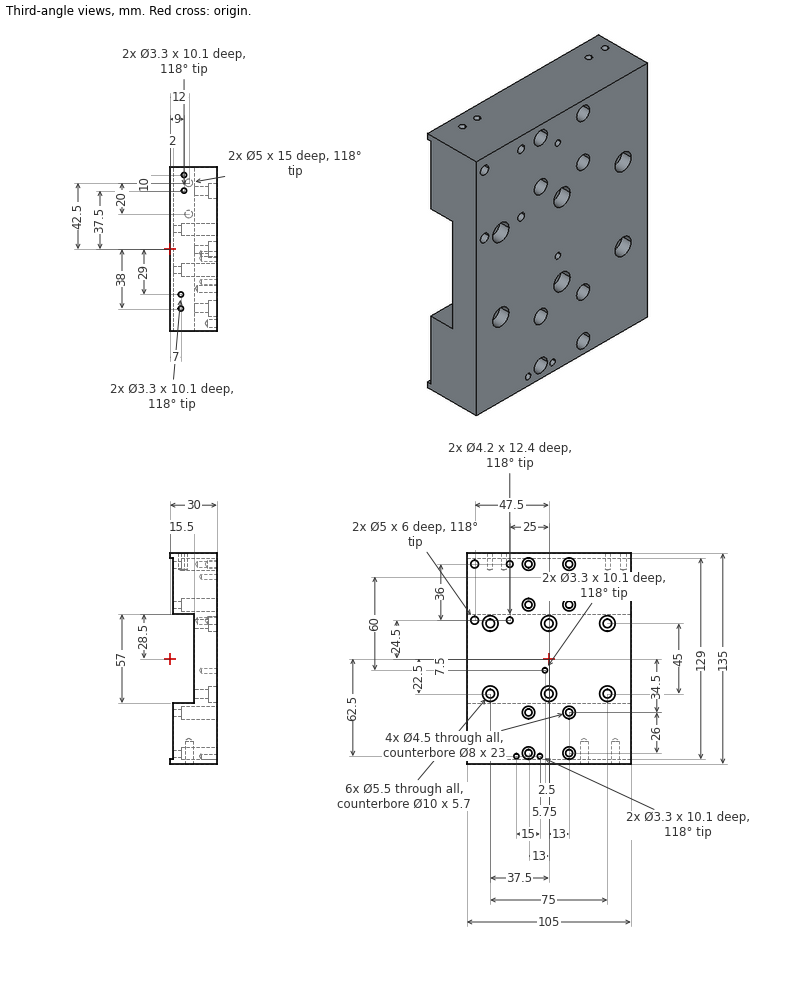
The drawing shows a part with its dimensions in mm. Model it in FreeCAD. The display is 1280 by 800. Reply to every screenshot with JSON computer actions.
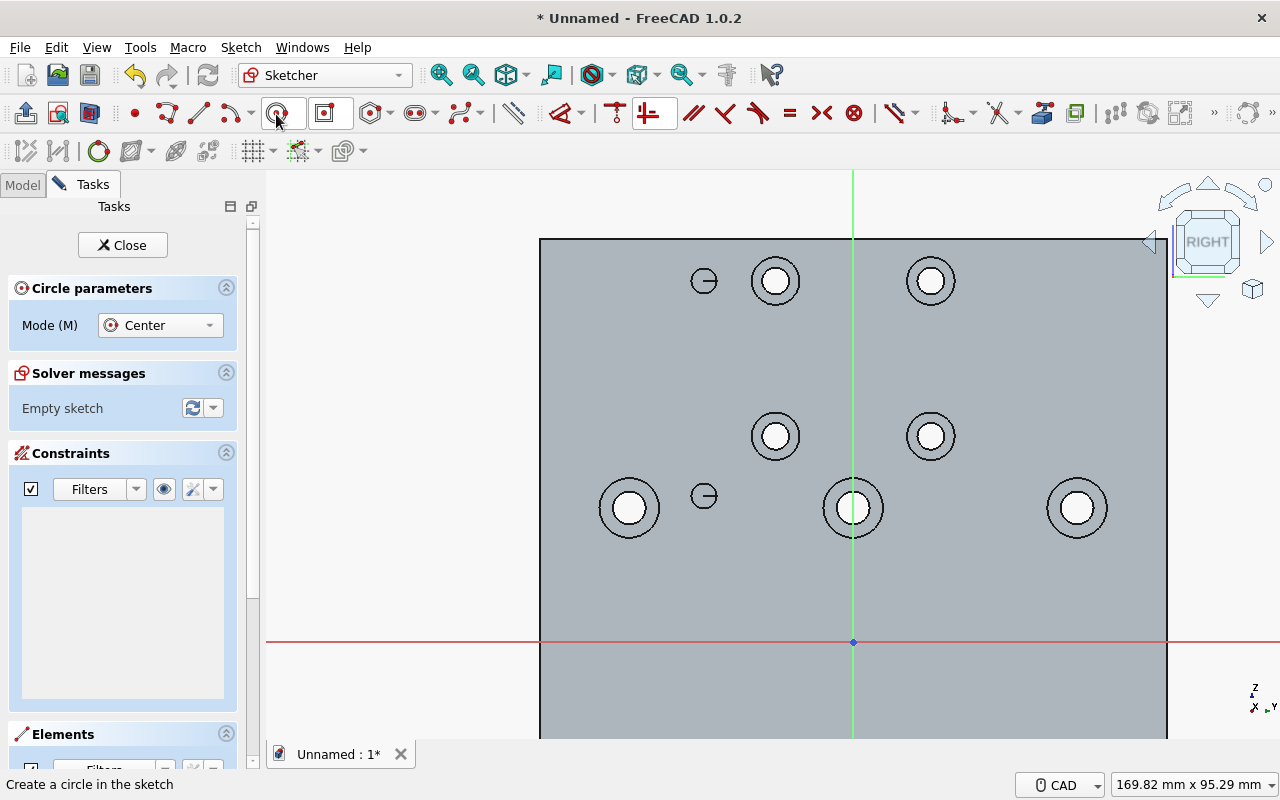
{"action": "scroll", "coordinate": [570, 496], "scroll_direction": "up", "scroll_amount": 3}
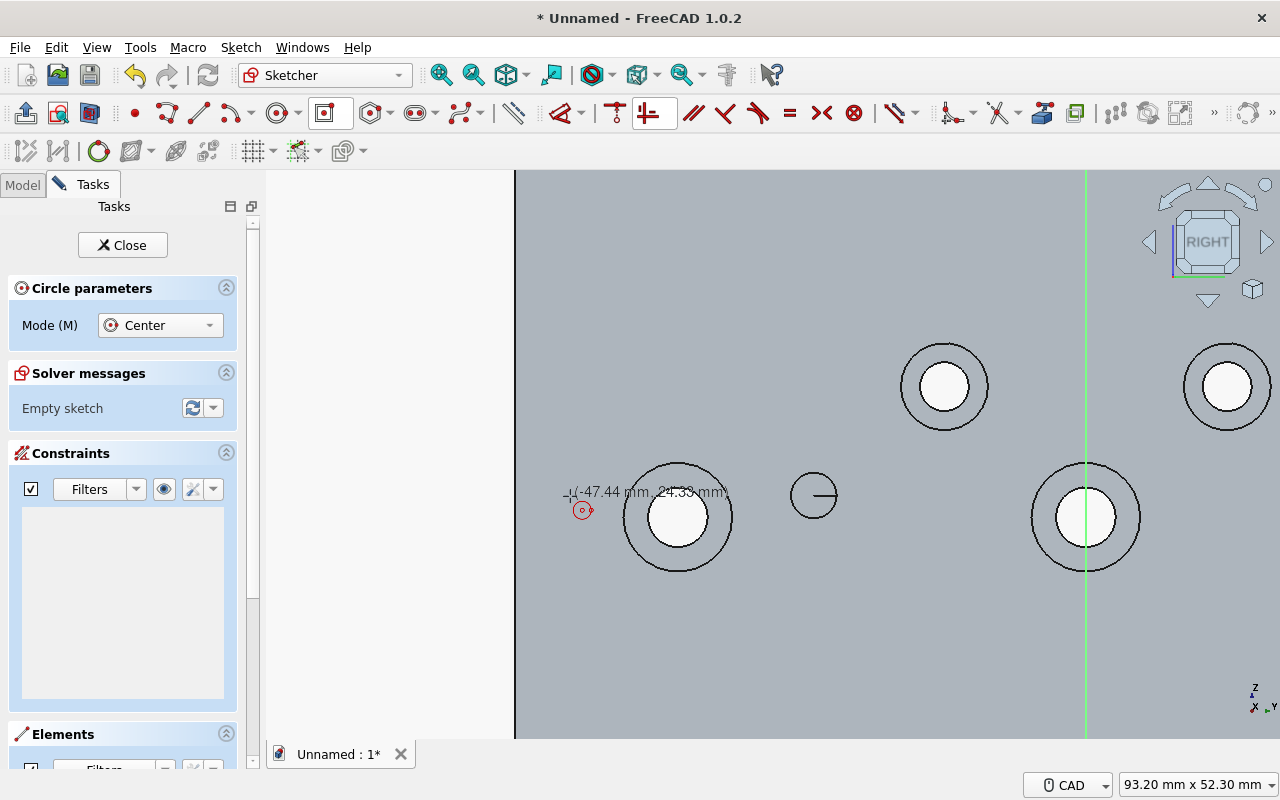
{"action": "left_click", "coordinate": [569, 495]}
{"action": "left_click", "coordinate": [588, 476]}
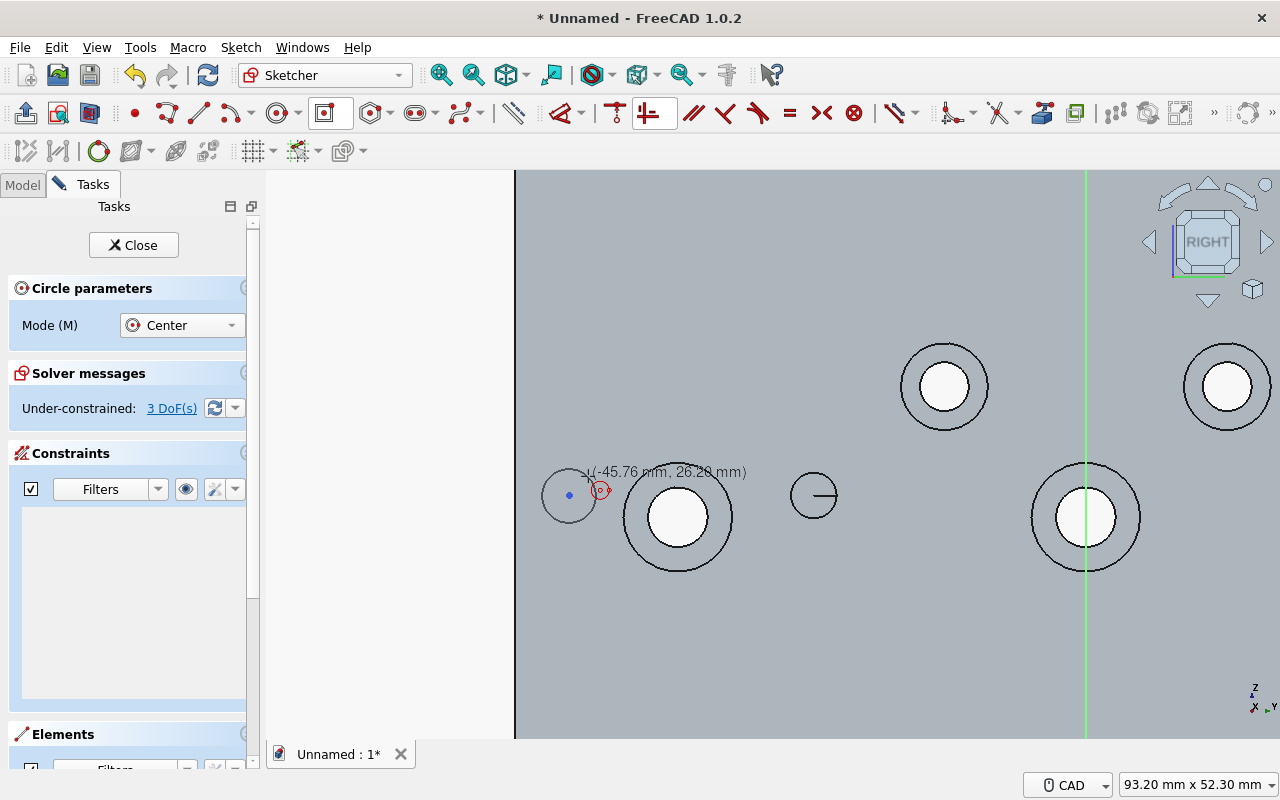
{"action": "scroll", "coordinate": [571, 497], "scroll_direction": "down", "scroll_amount": 3}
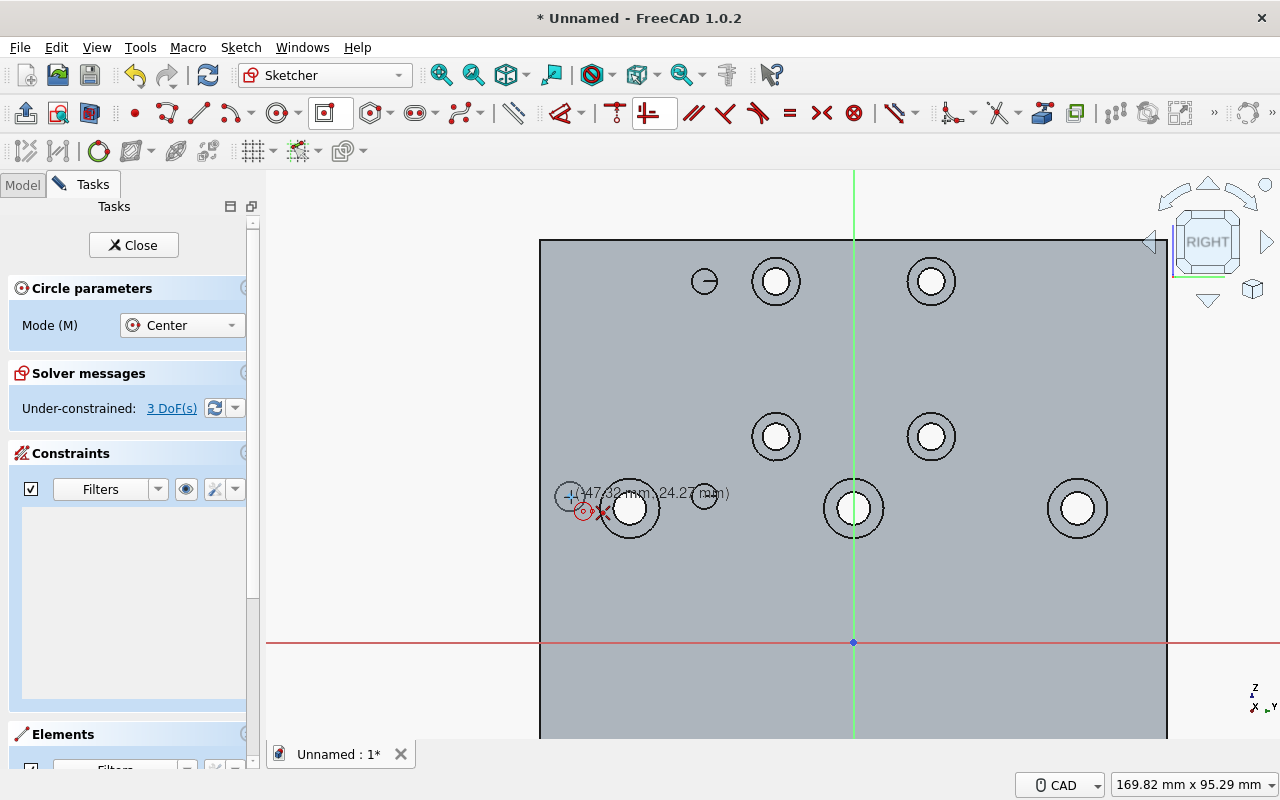
{"action": "scroll", "coordinate": [570, 281], "scroll_direction": "up", "scroll_amount": 3}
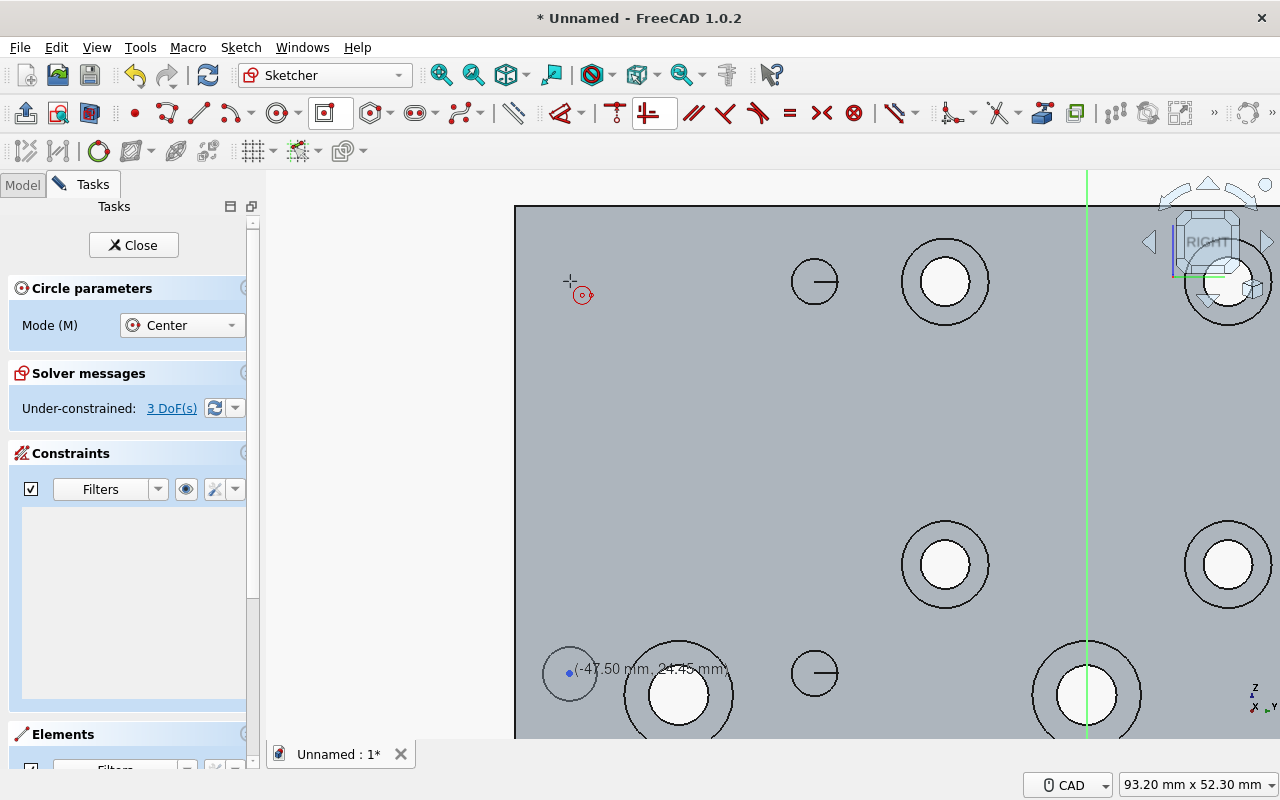
{"action": "left_click", "coordinate": [570, 282]}
{"action": "left_click", "coordinate": [589, 262]}
{"action": "key", "text": "Escape"}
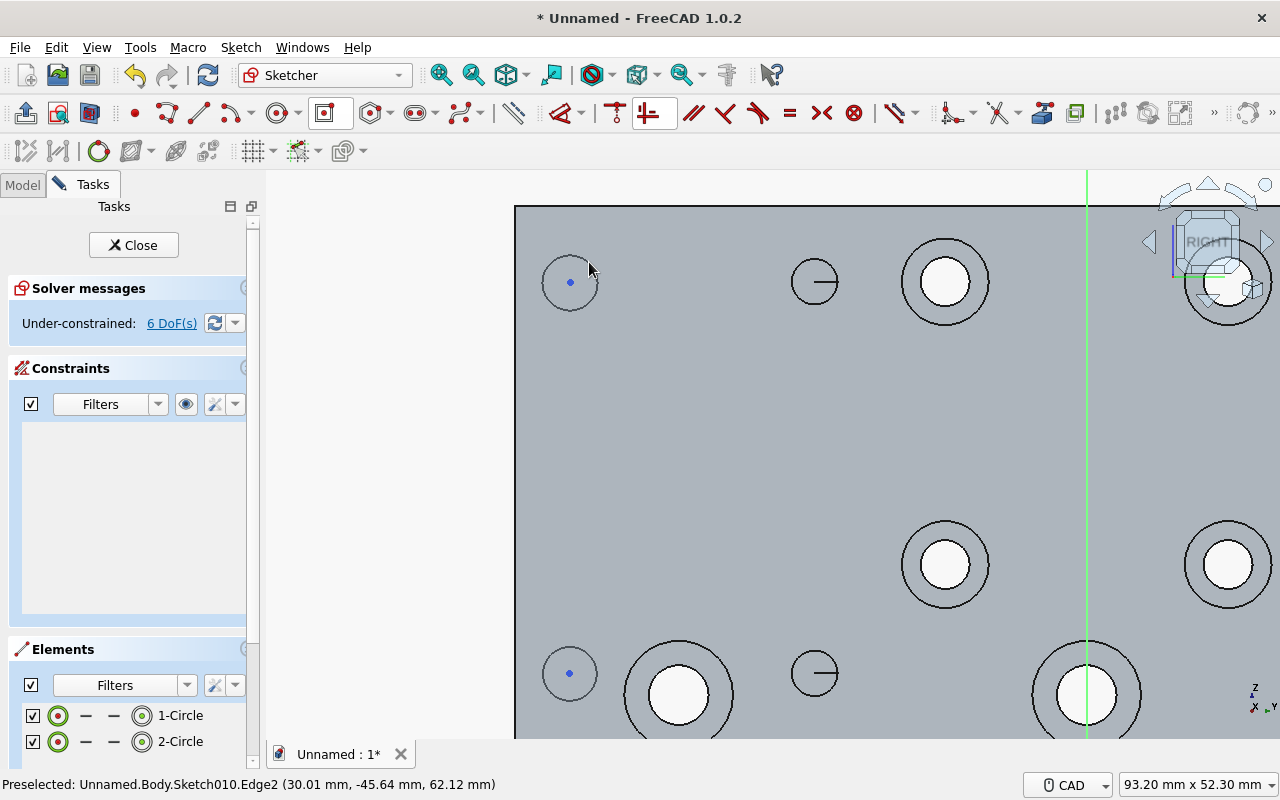
{"action": "left_click", "coordinate": [589, 655]}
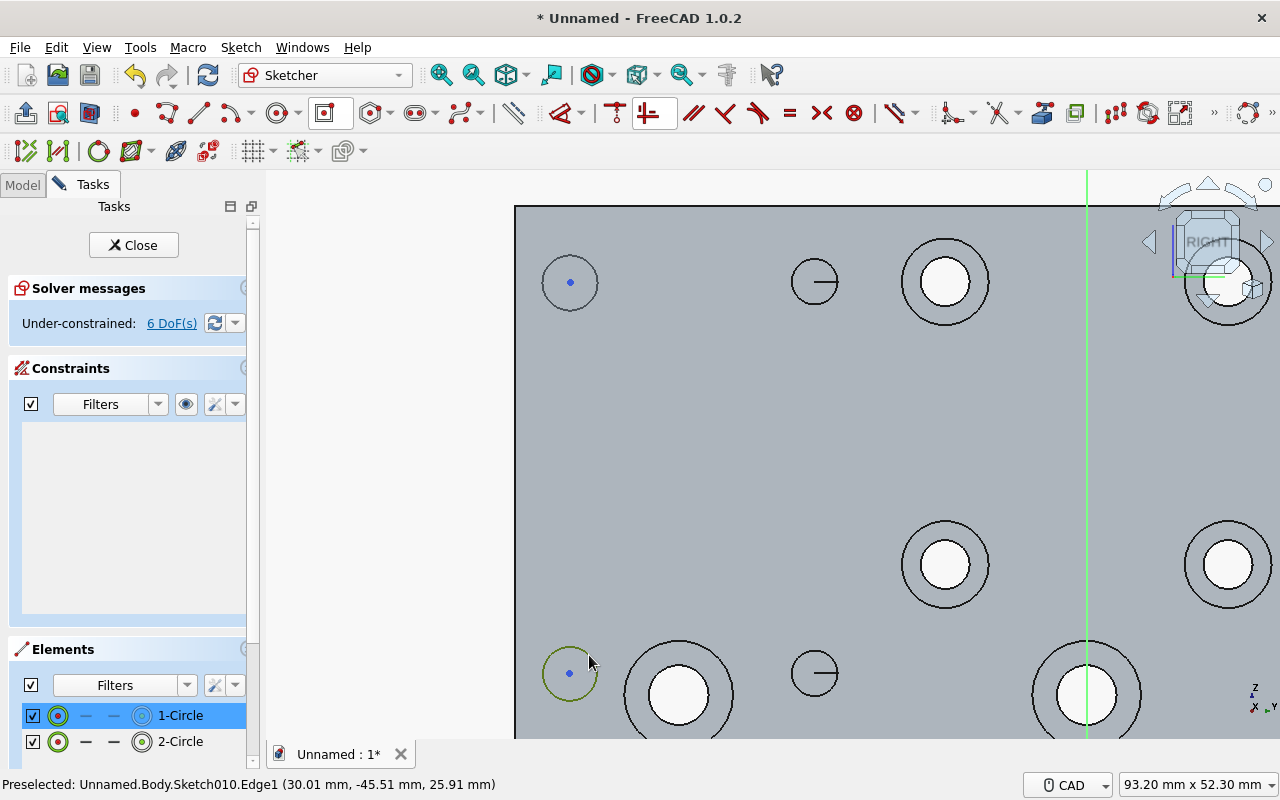
{"action": "left_click", "coordinate": [589, 263]}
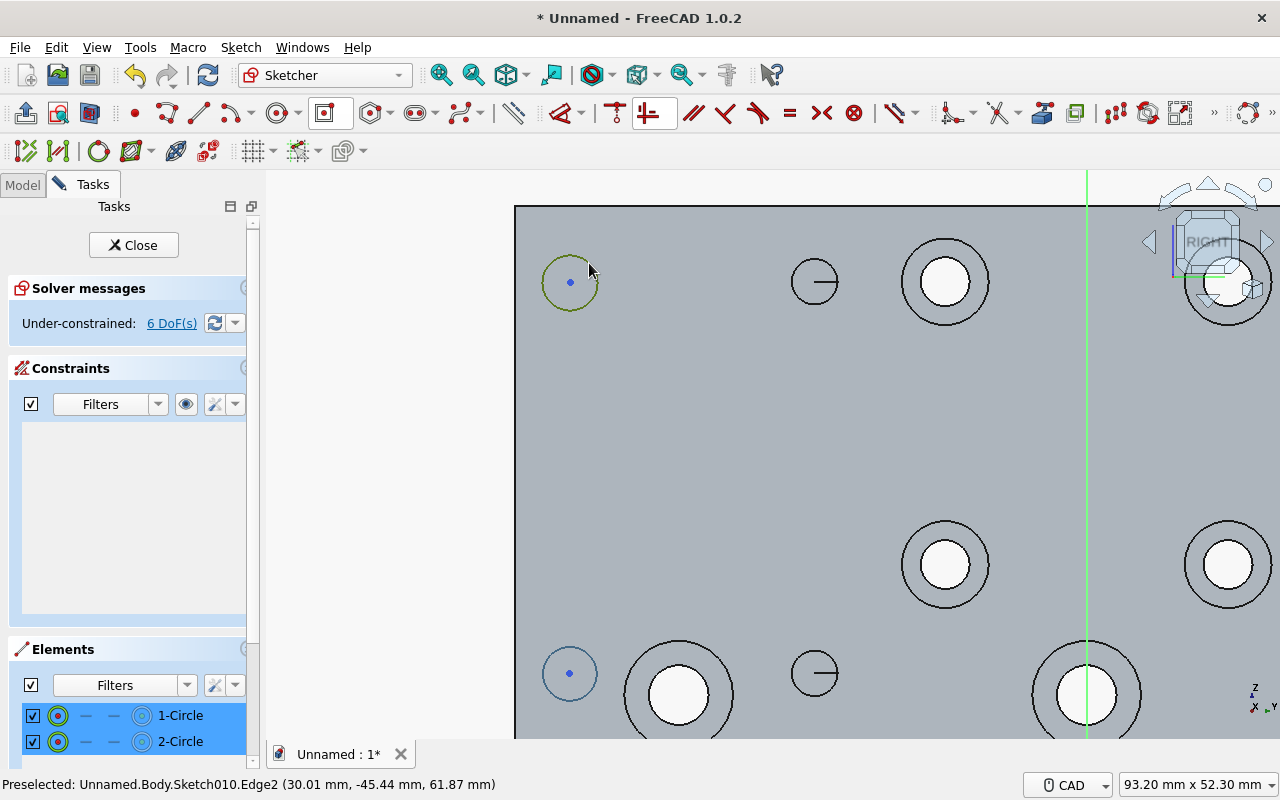
{"action": "left_click", "coordinate": [790, 114]}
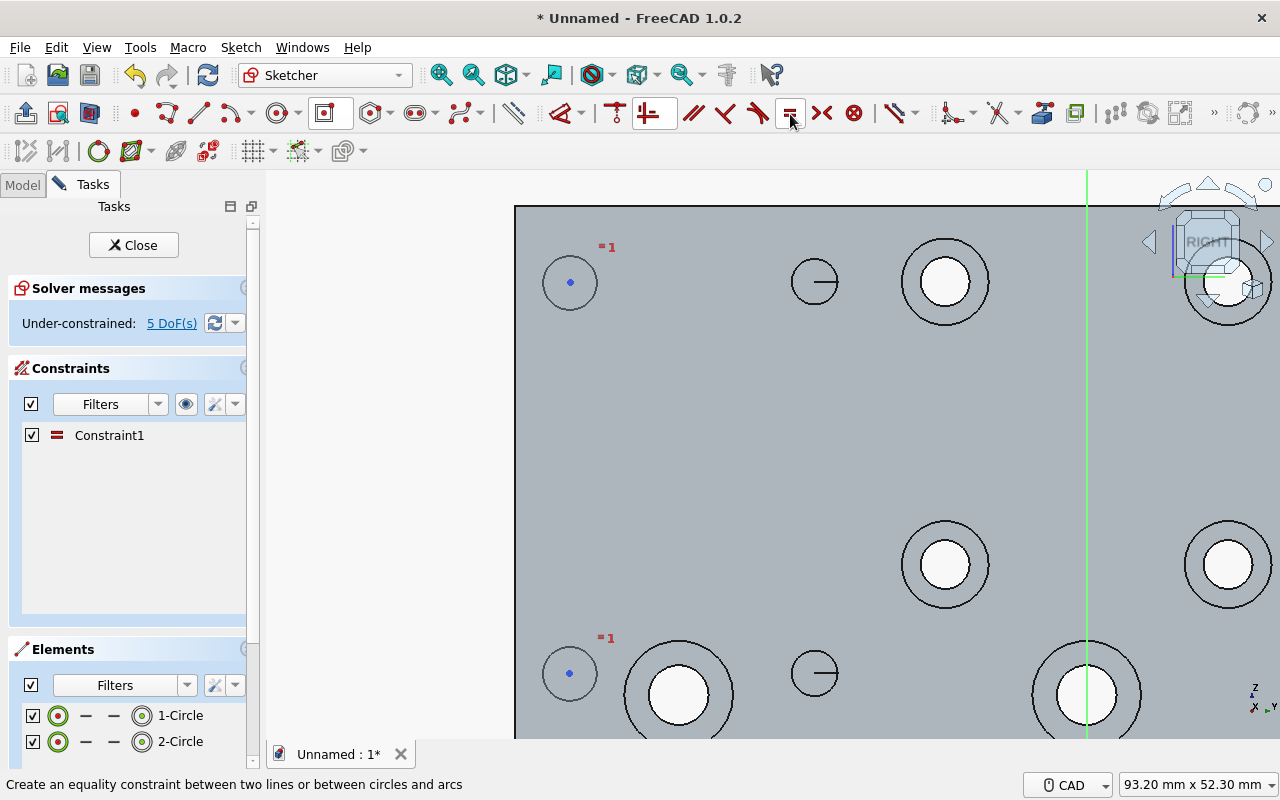
{"action": "left_click", "coordinate": [570, 674]}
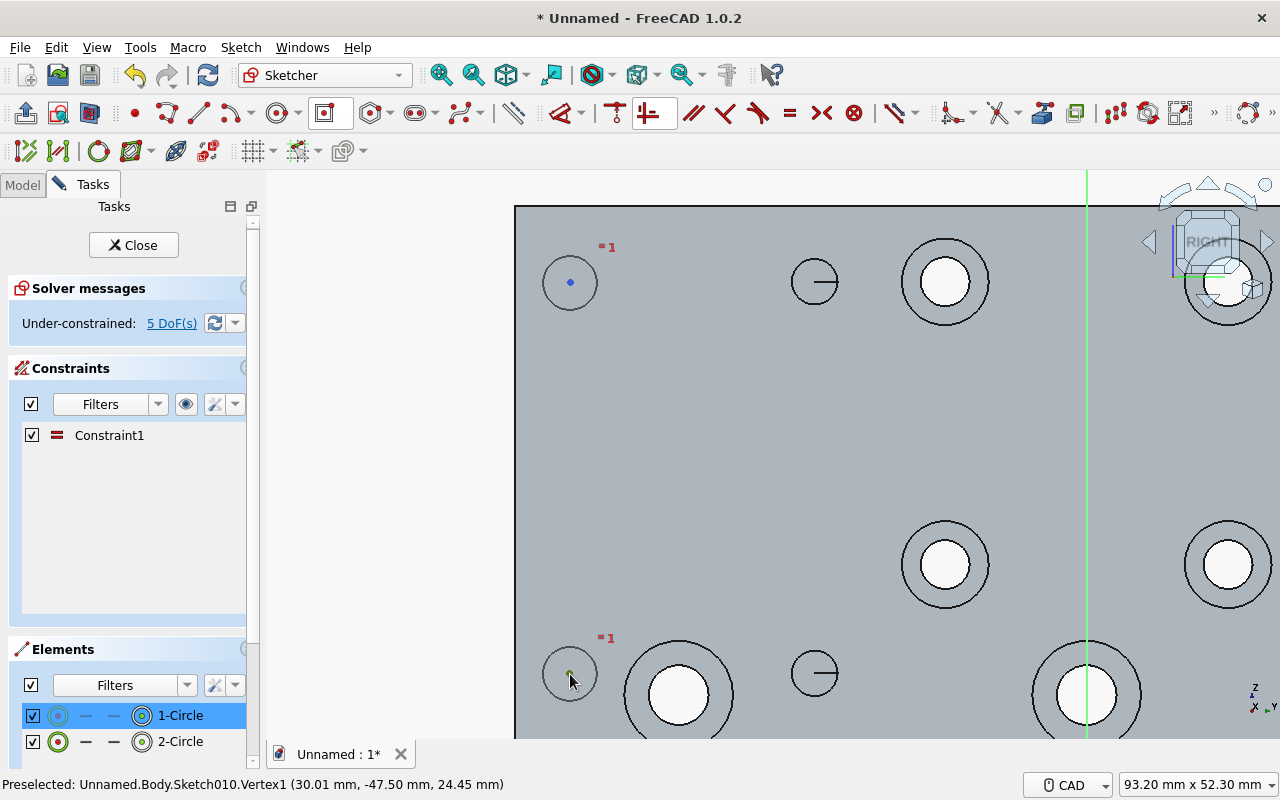
{"action": "left_click", "coordinate": [570, 283]}